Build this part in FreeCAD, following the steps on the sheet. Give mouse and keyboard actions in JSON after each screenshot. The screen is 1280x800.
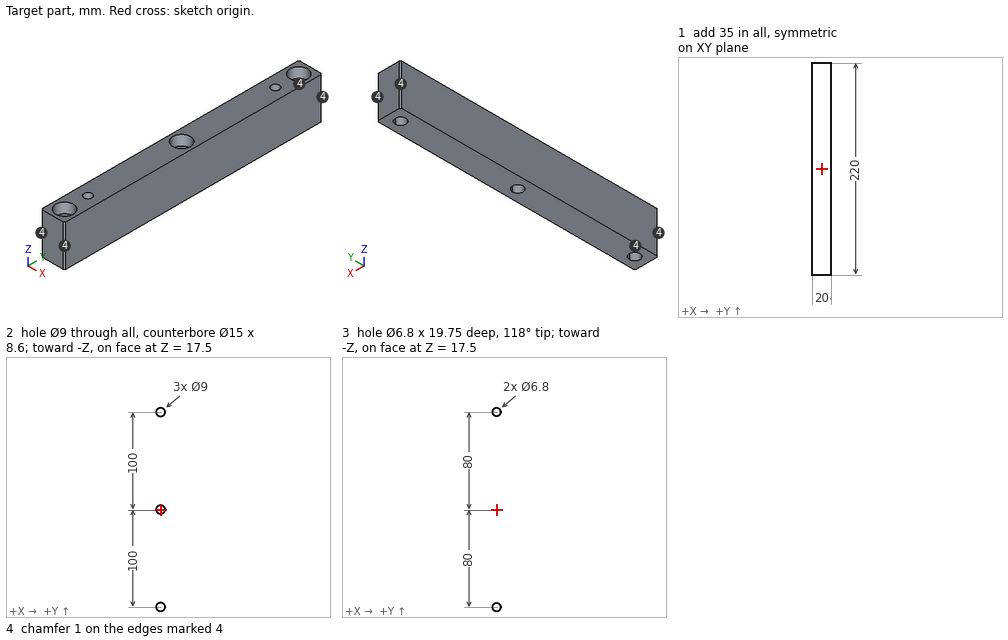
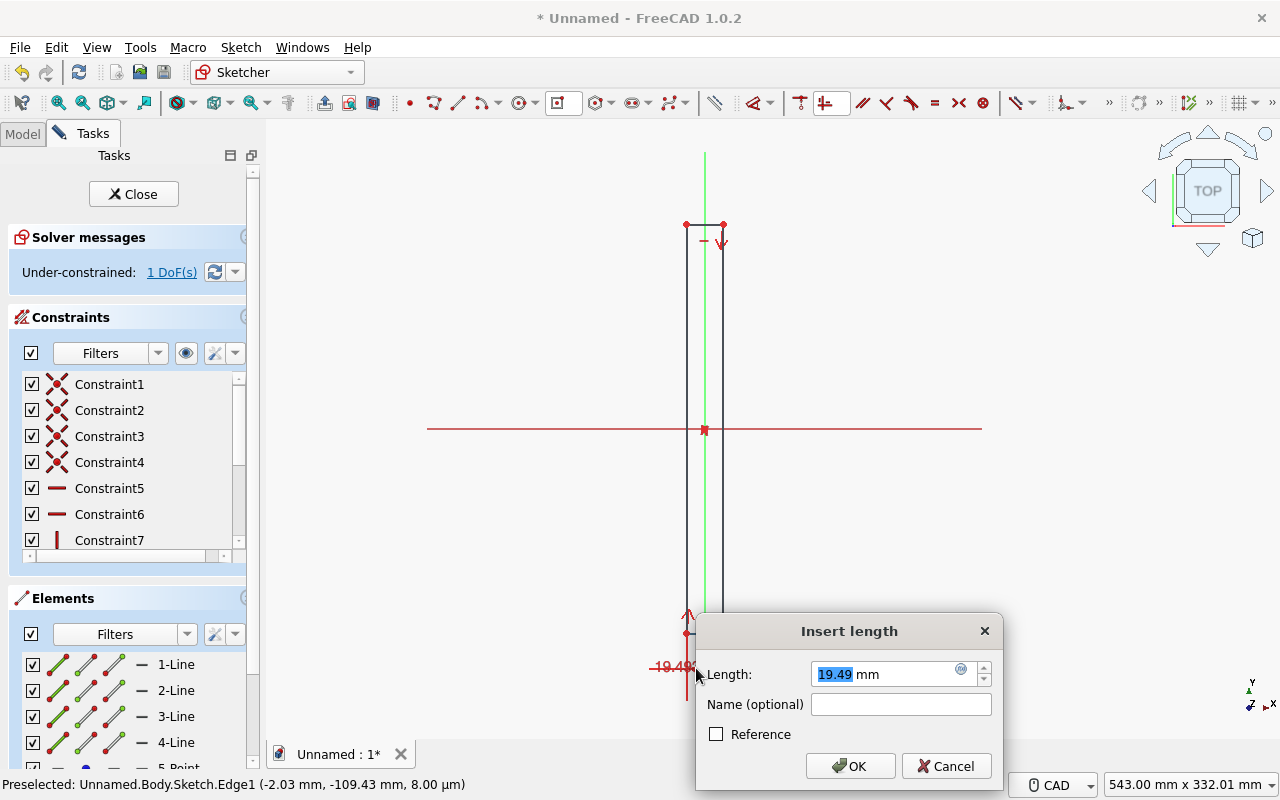
{"action": "type", "text": "20"}
{"action": "key", "text": "Return"}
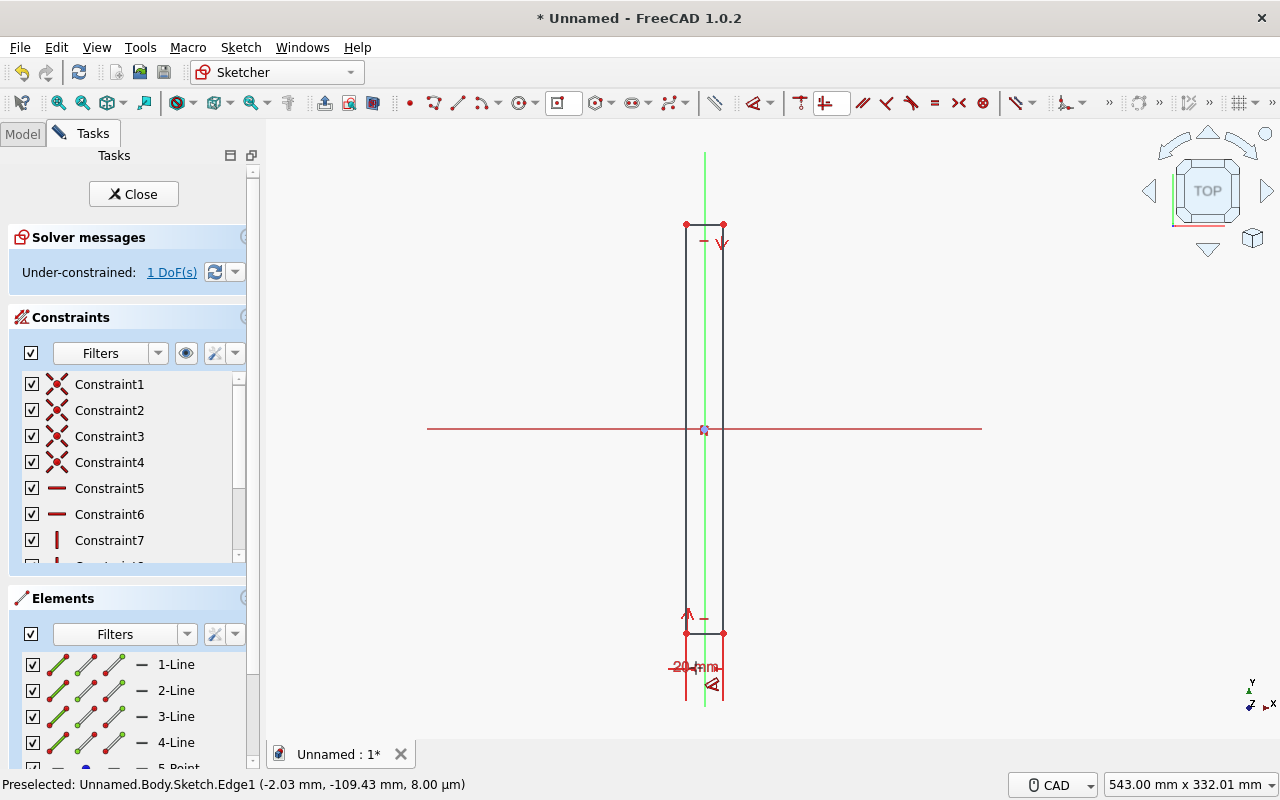
{"action": "left_click", "coordinate": [723, 511]}
{"action": "left_click", "coordinate": [757, 335]}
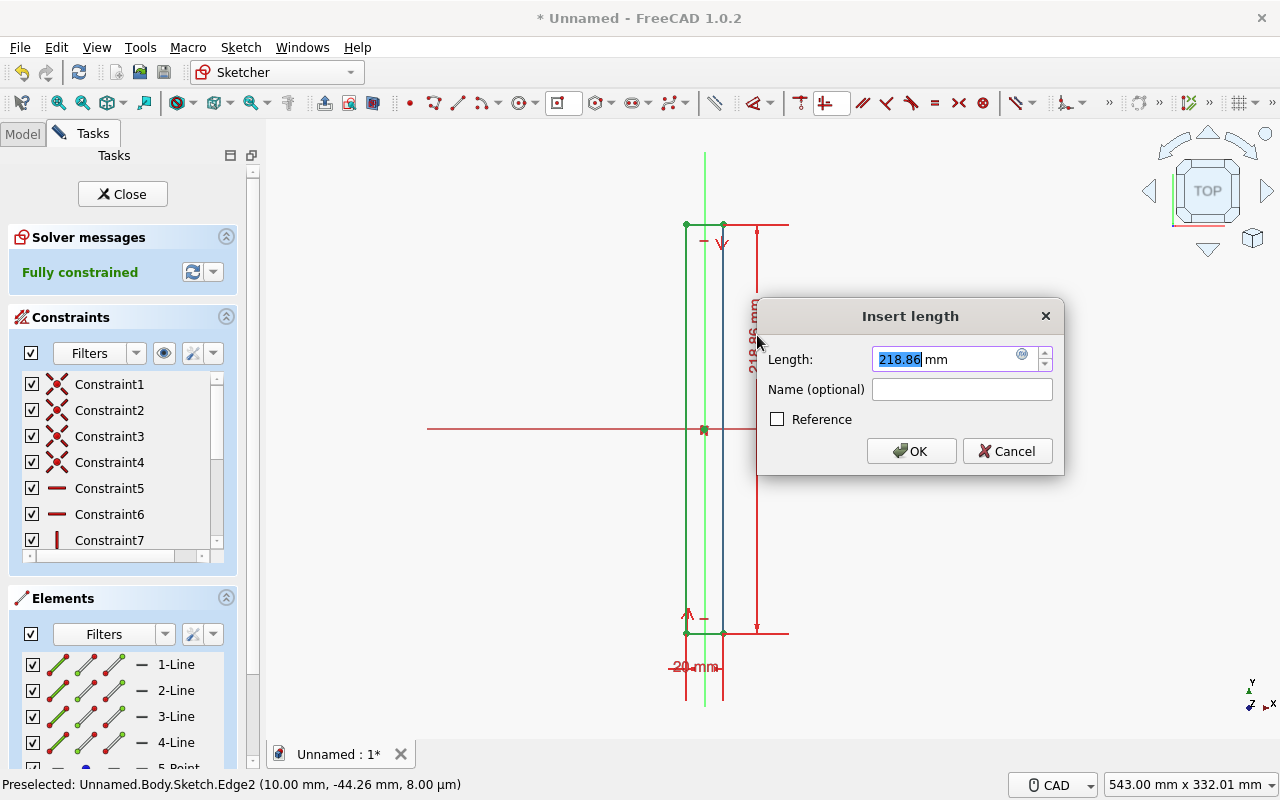
{"action": "type", "text": "220"}
{"action": "key", "text": "Return"}
{"action": "key", "text": "Escape"}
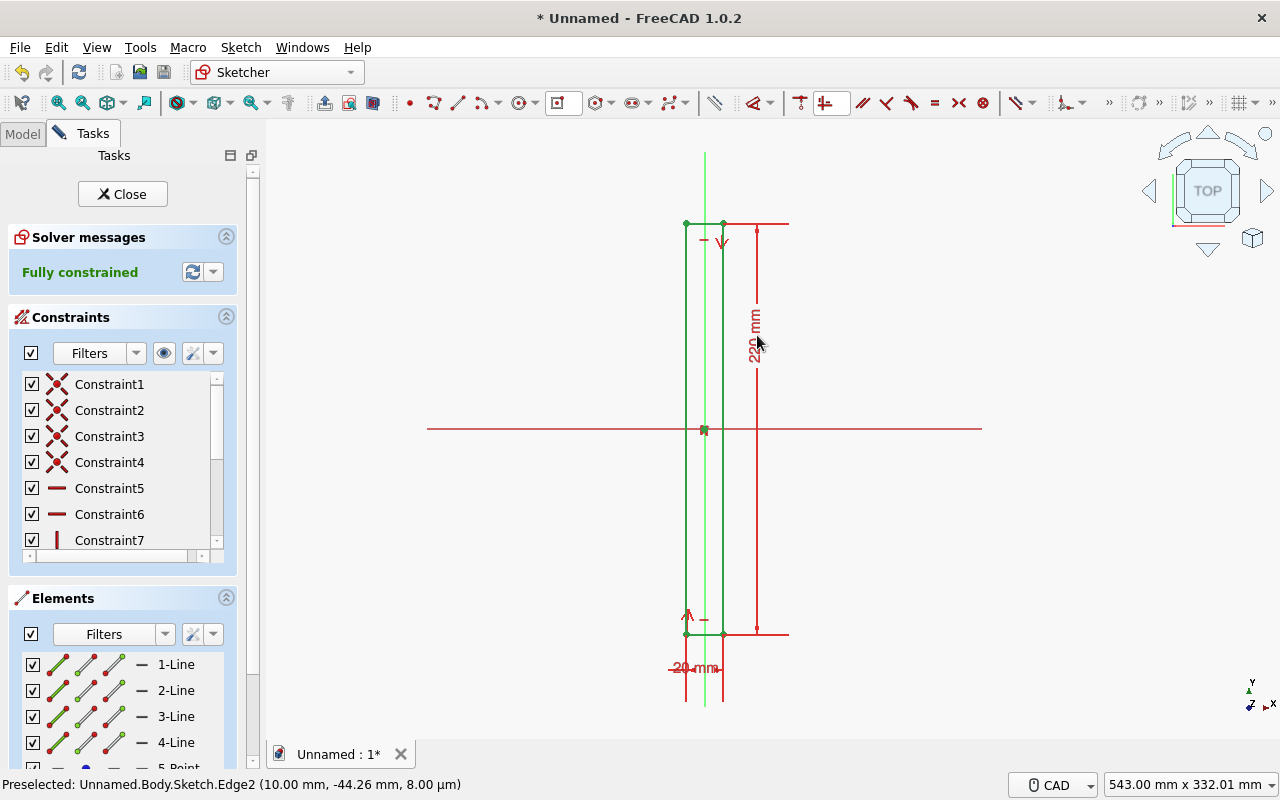
{"action": "left_click", "coordinate": [123, 194]}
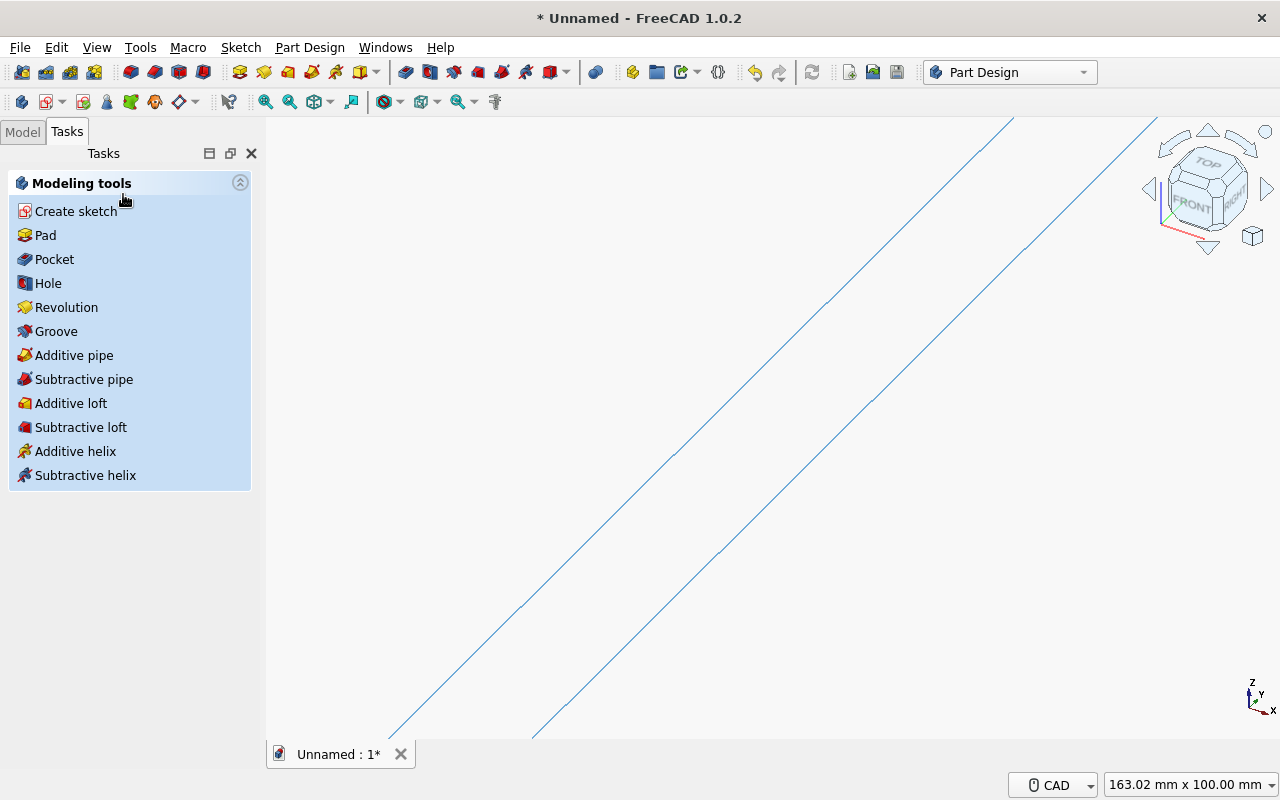
{"action": "left_click", "coordinate": [240, 72]}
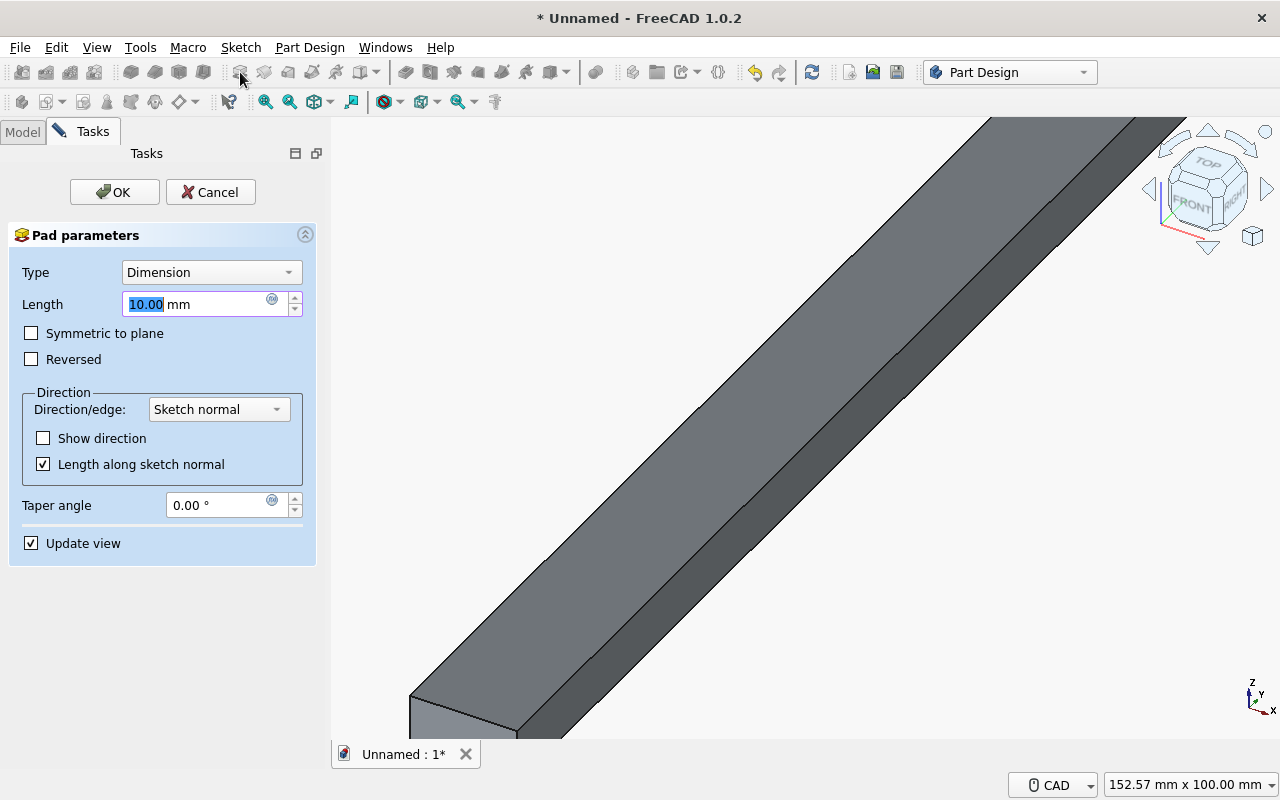
{"action": "type", "text": "35"}
{"action": "key", "text": "Tab"}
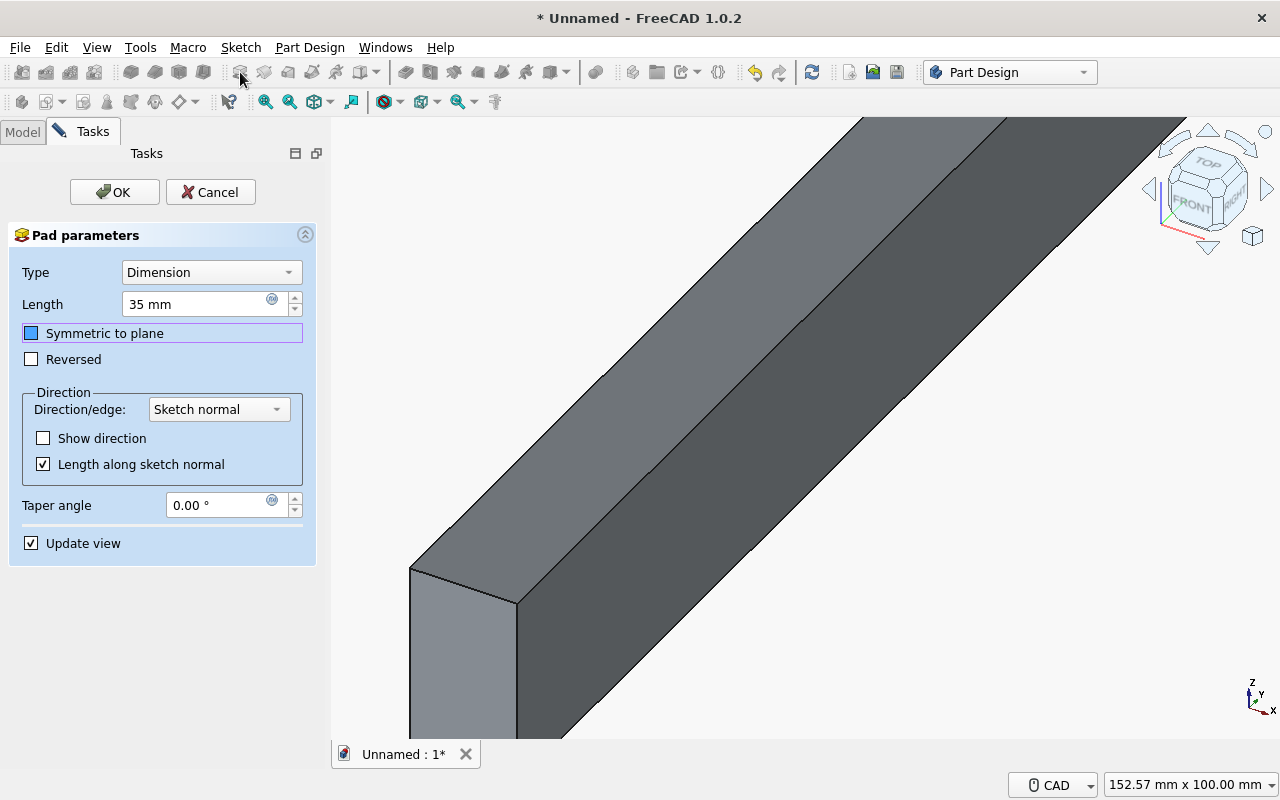
{"action": "left_click", "coordinate": [30, 333]}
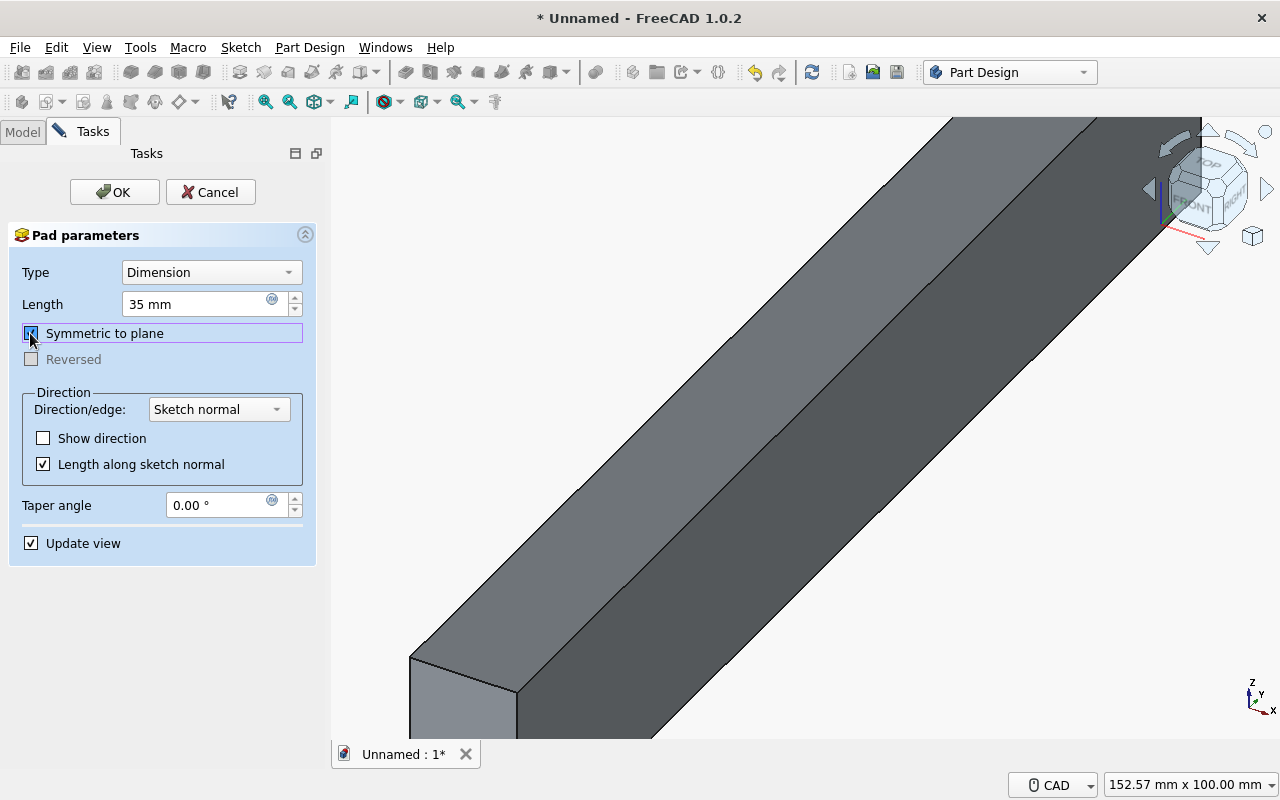
{"action": "left_click", "coordinate": [115, 192]}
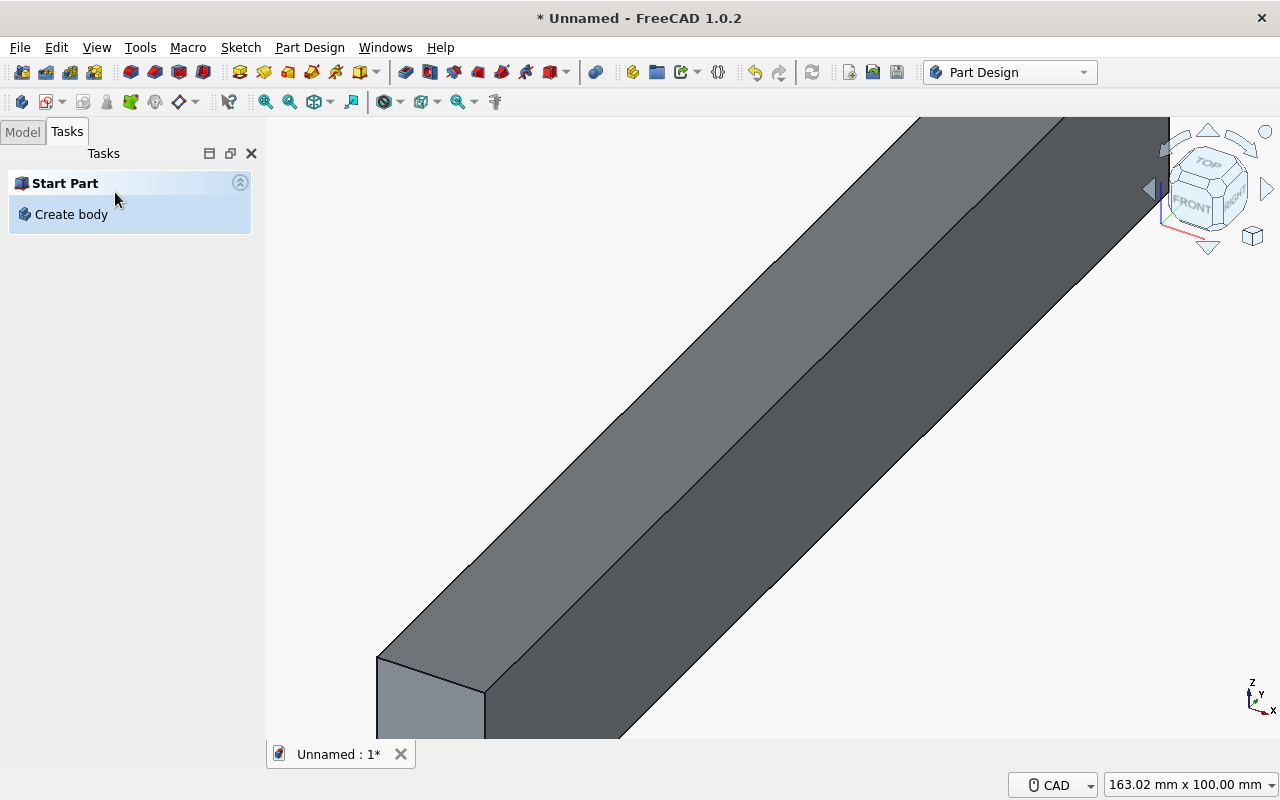
{"action": "left_click", "coordinate": [266, 102]}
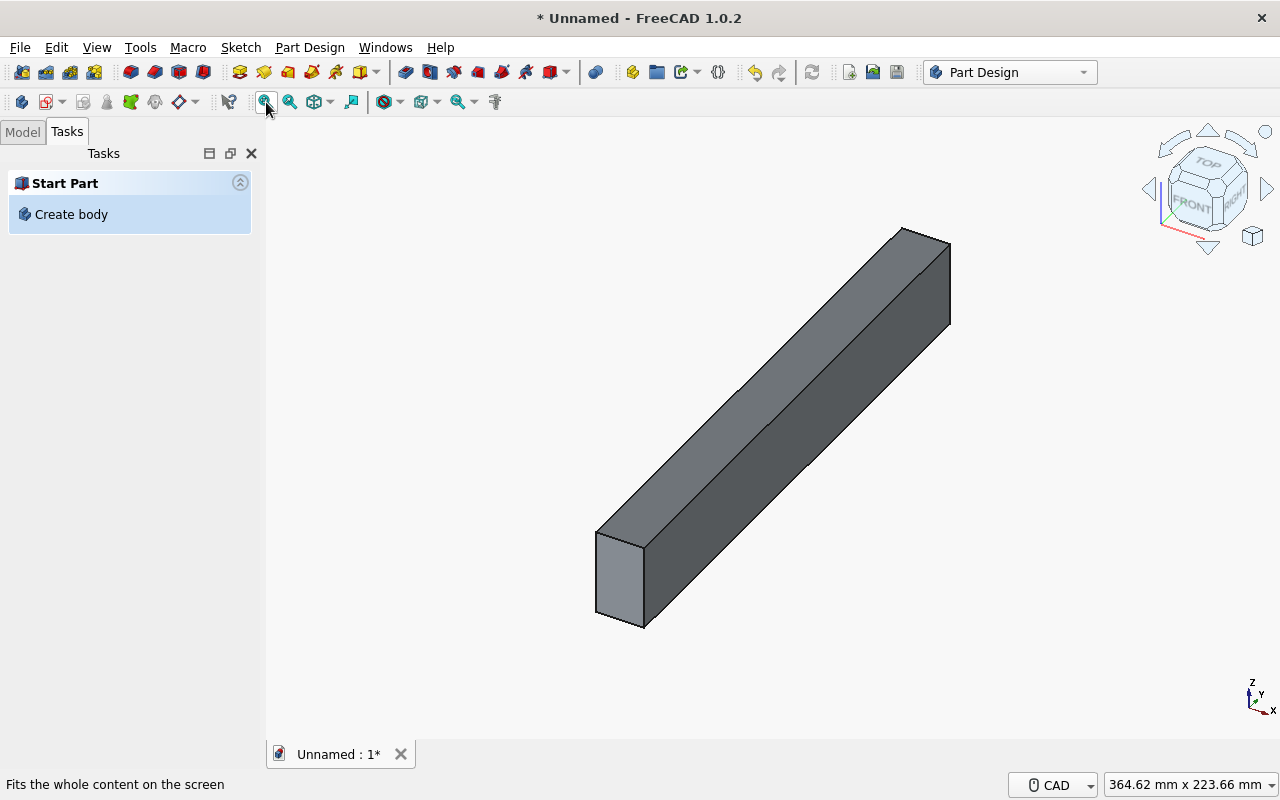
{"action": "left_click", "coordinate": [904, 257]}